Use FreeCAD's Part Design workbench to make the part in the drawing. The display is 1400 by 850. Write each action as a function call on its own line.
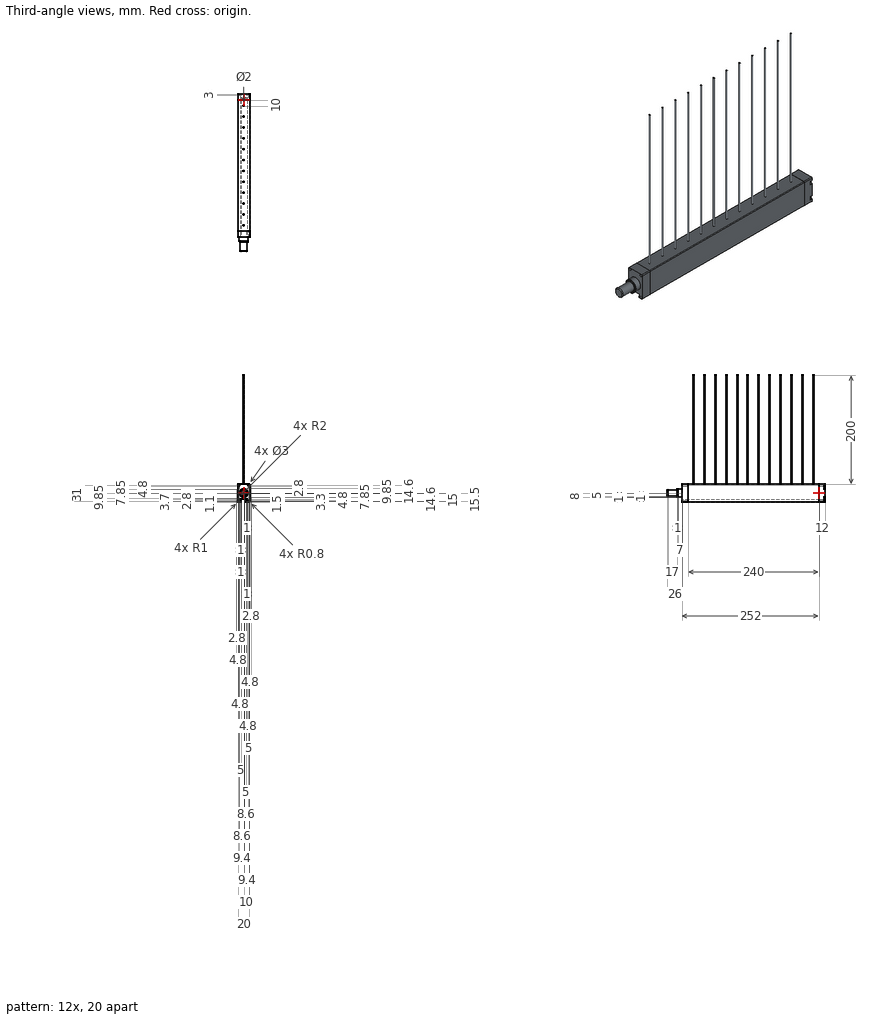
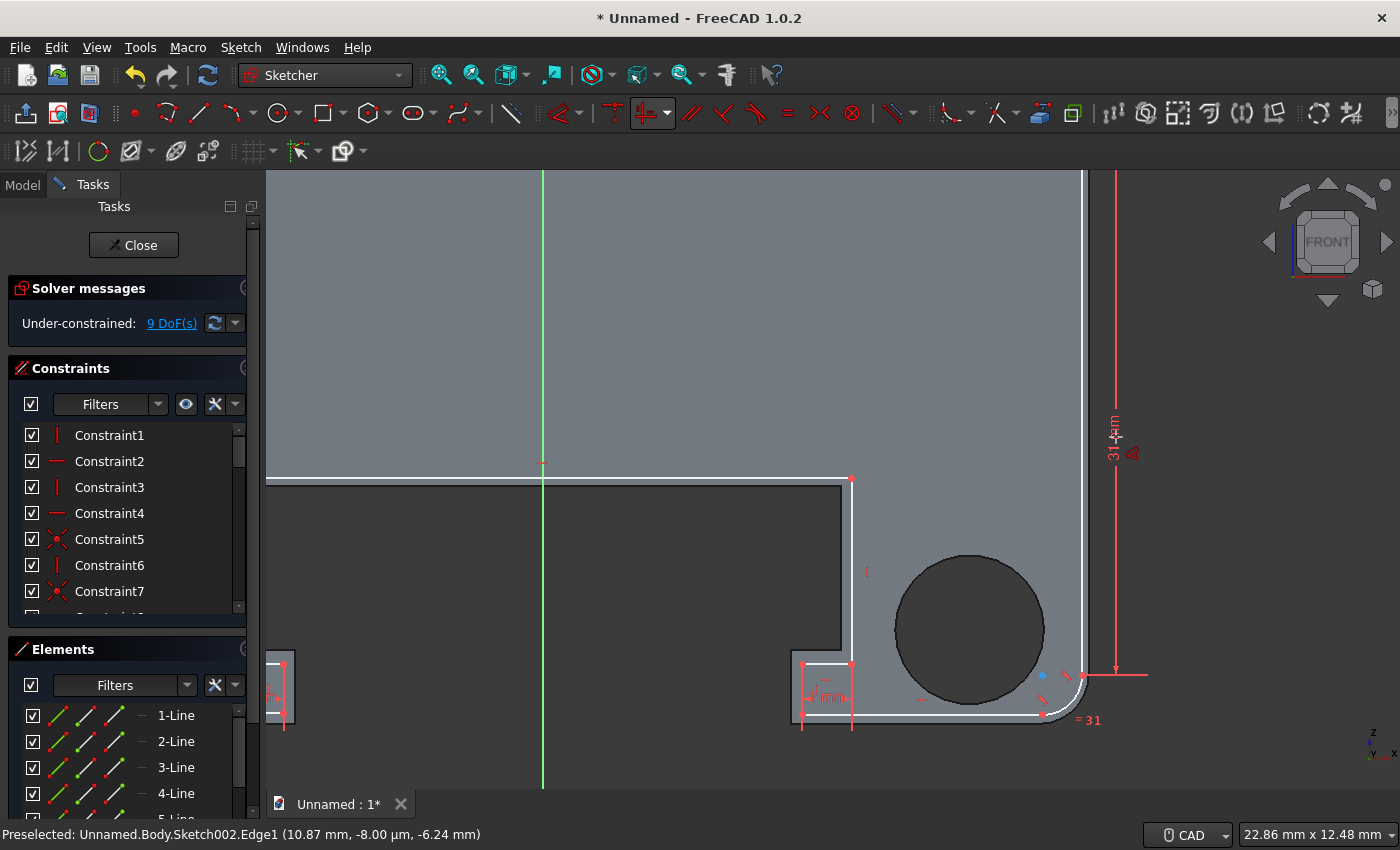
scroll(837, 667, down, 7)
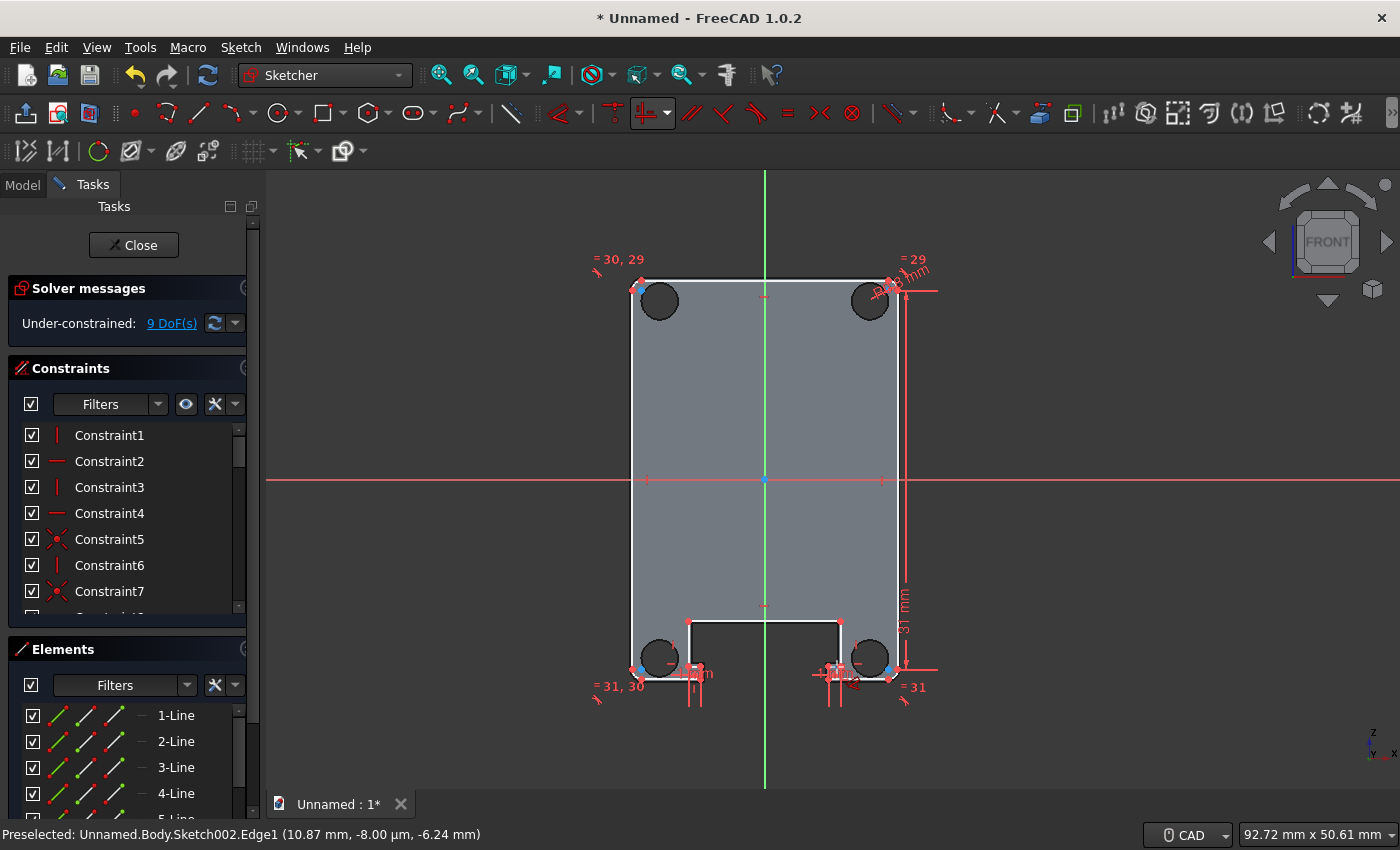
click(814, 281)
click(708, 247)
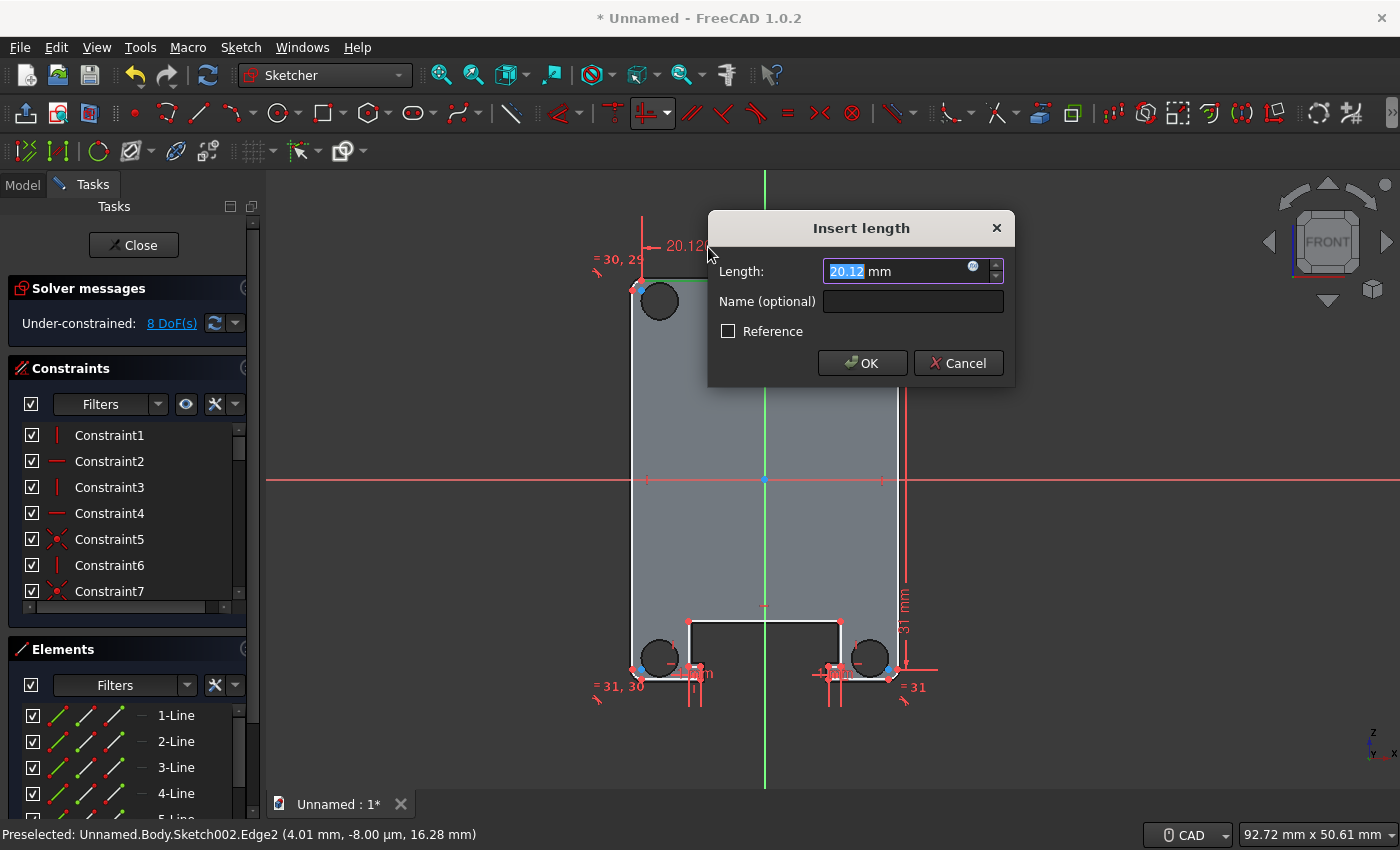
text(20)
key(Return)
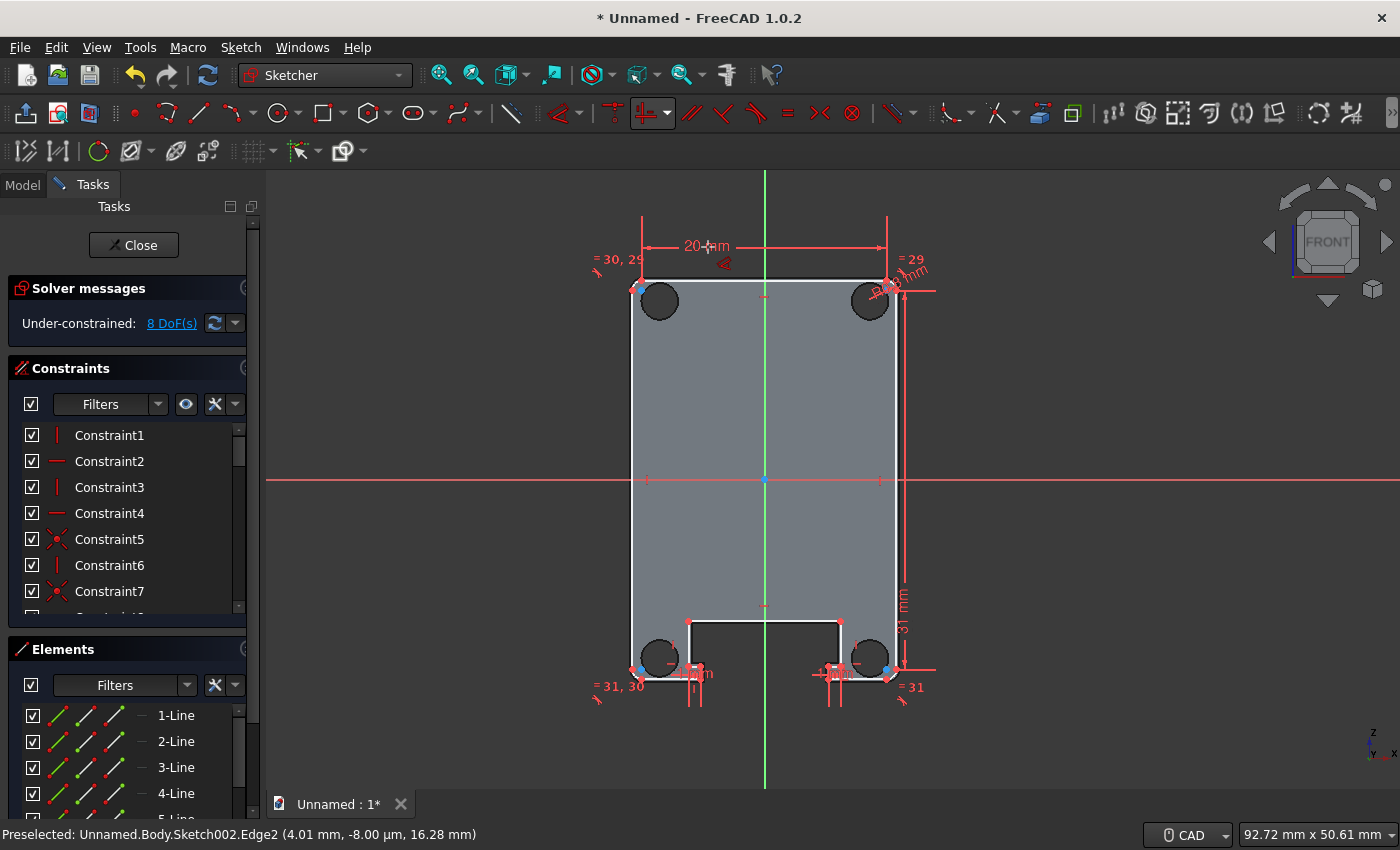
click(632, 404)
click(598, 393)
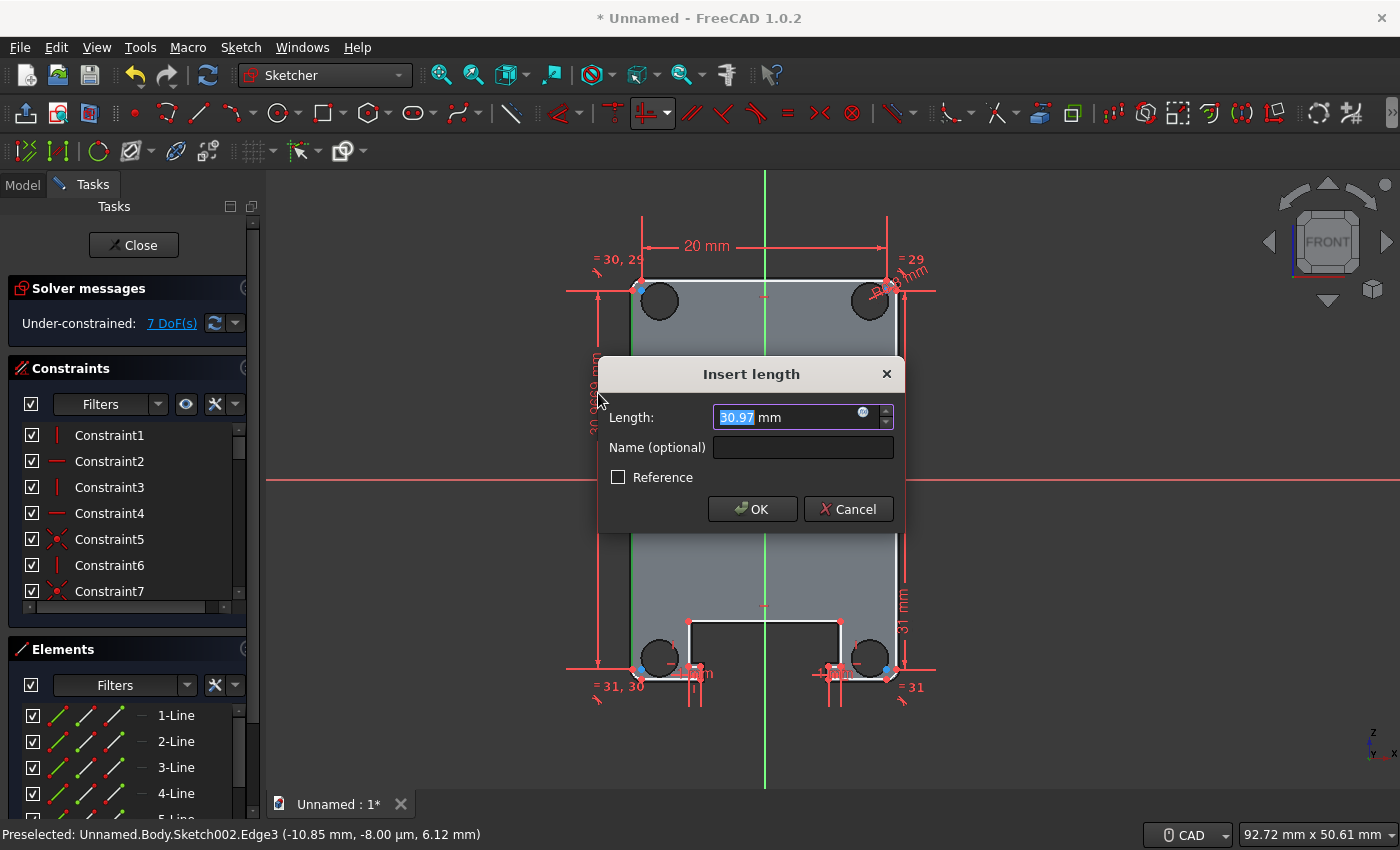
text(31)
key(Return)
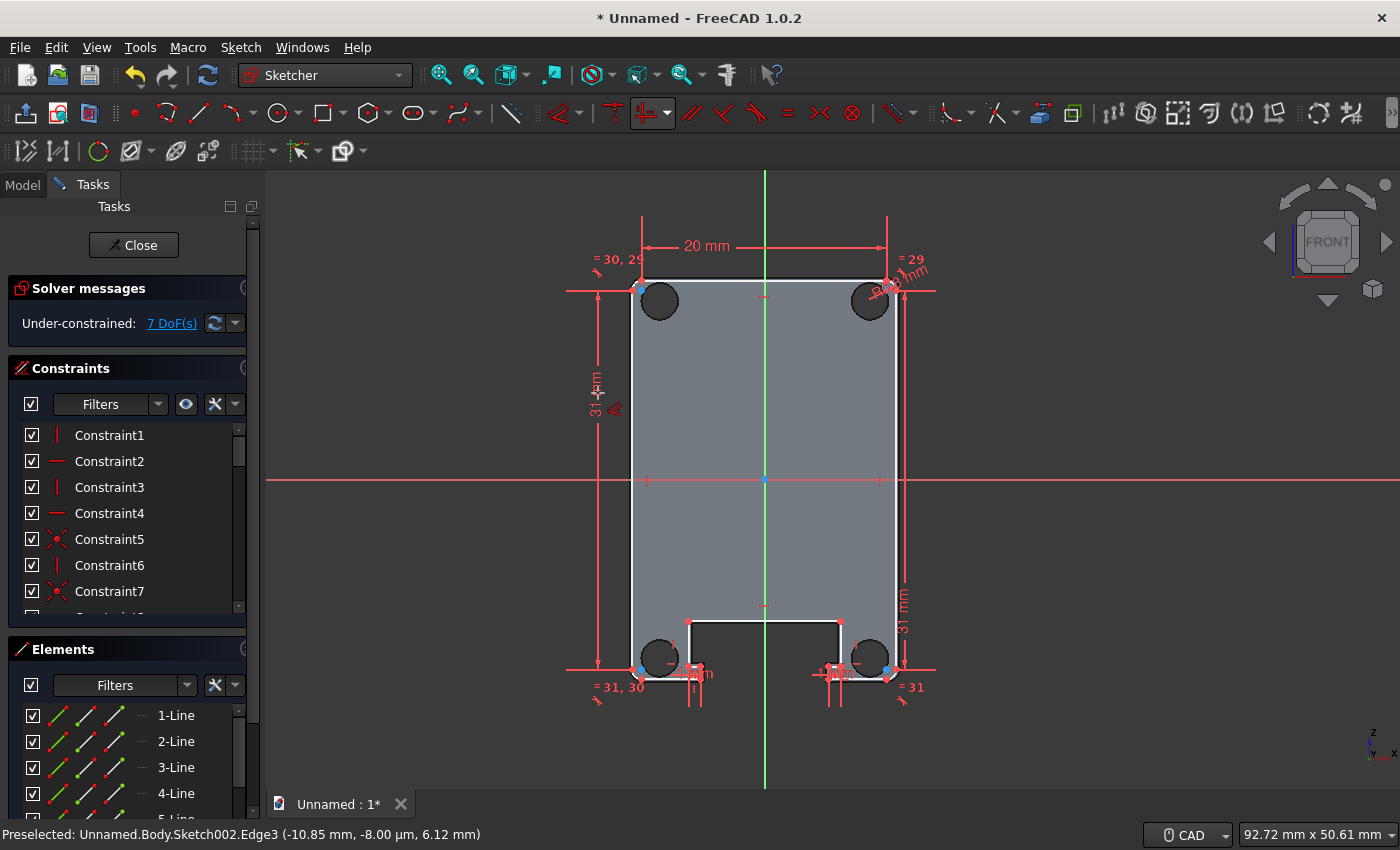
click(660, 679)
click(671, 713)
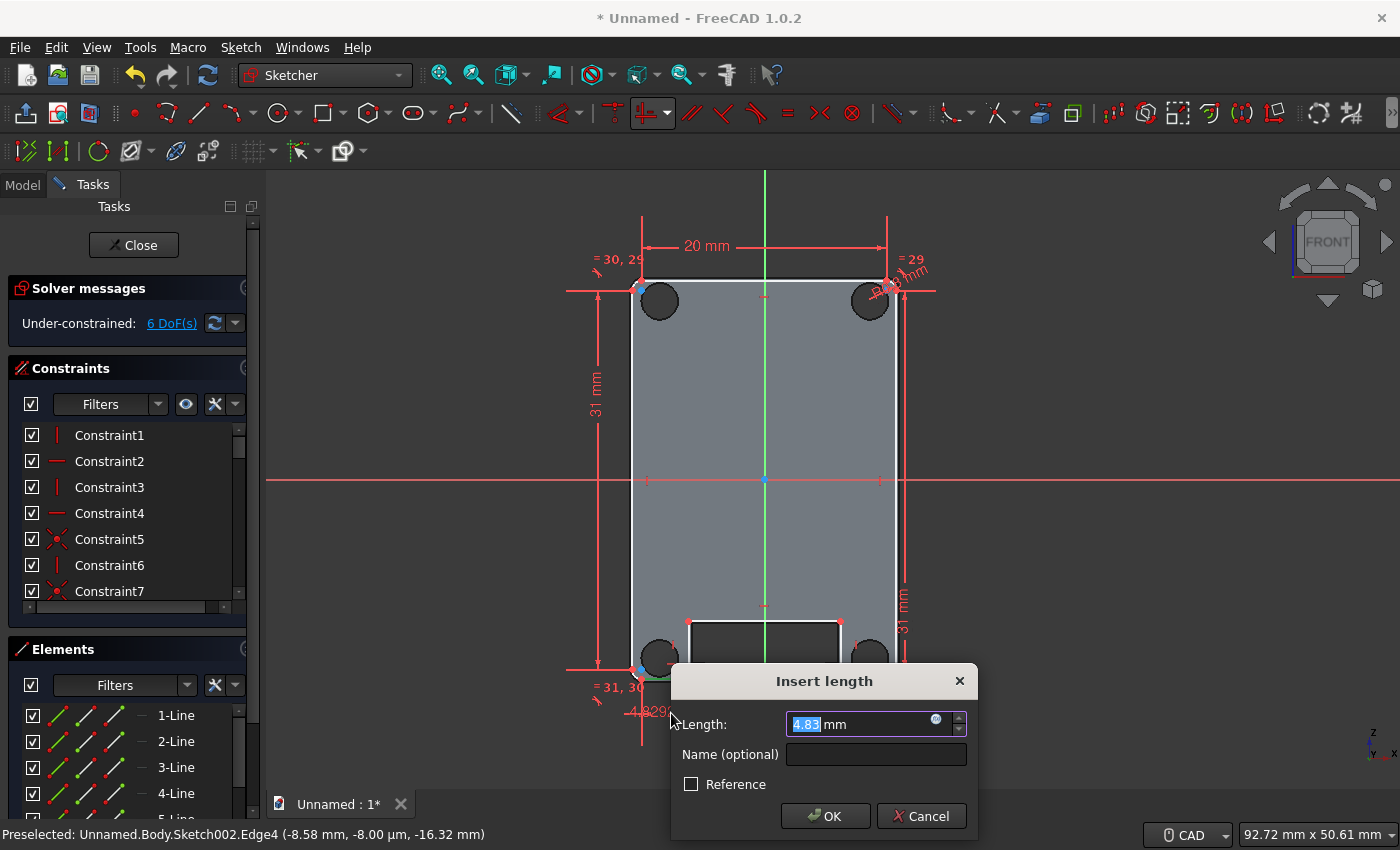
text(4.8)
key(Return)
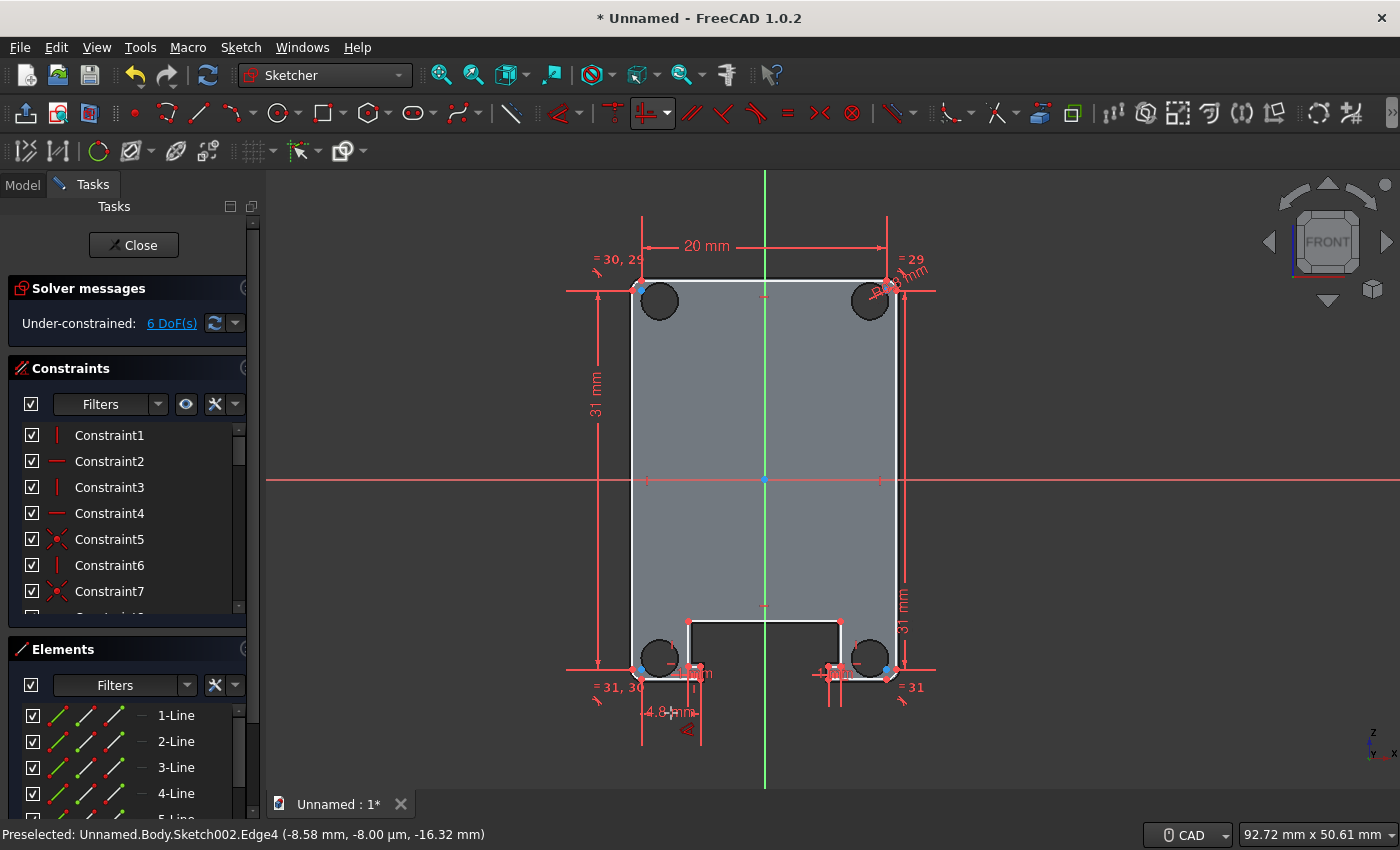
scroll(701, 673, up, 6)